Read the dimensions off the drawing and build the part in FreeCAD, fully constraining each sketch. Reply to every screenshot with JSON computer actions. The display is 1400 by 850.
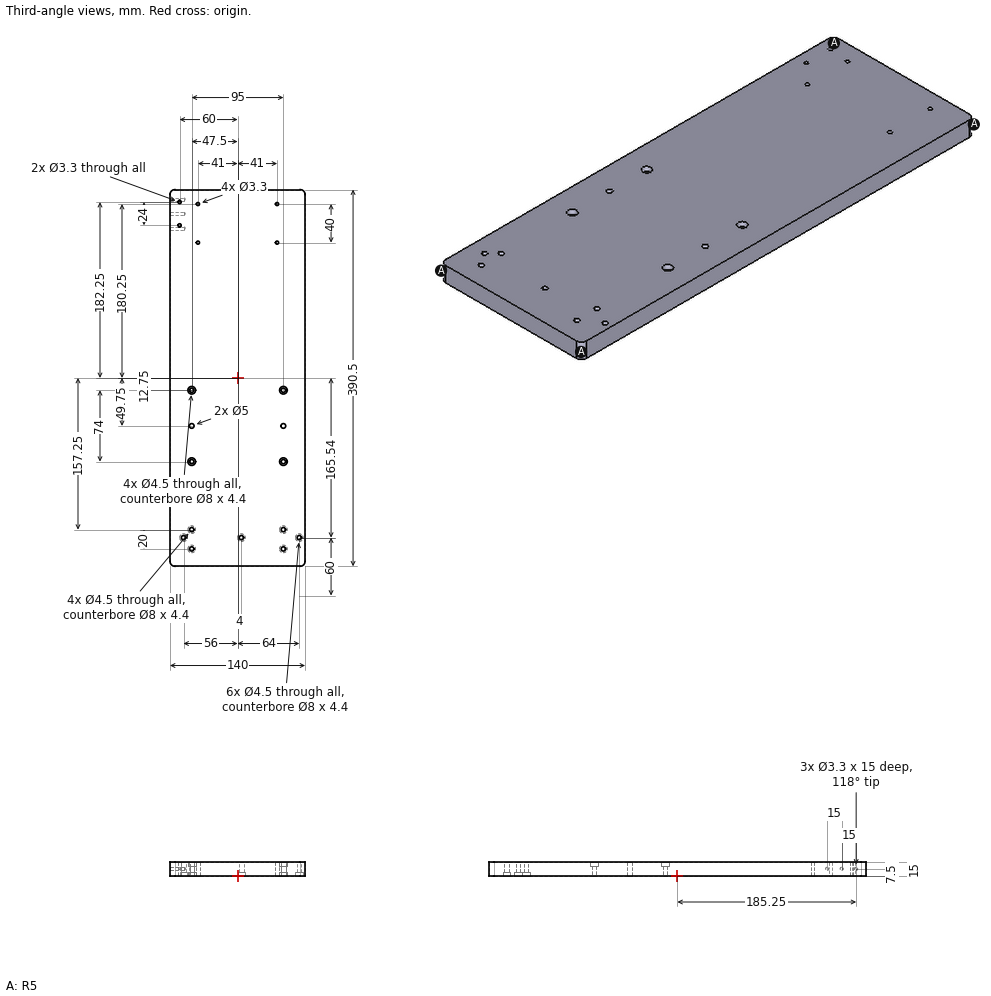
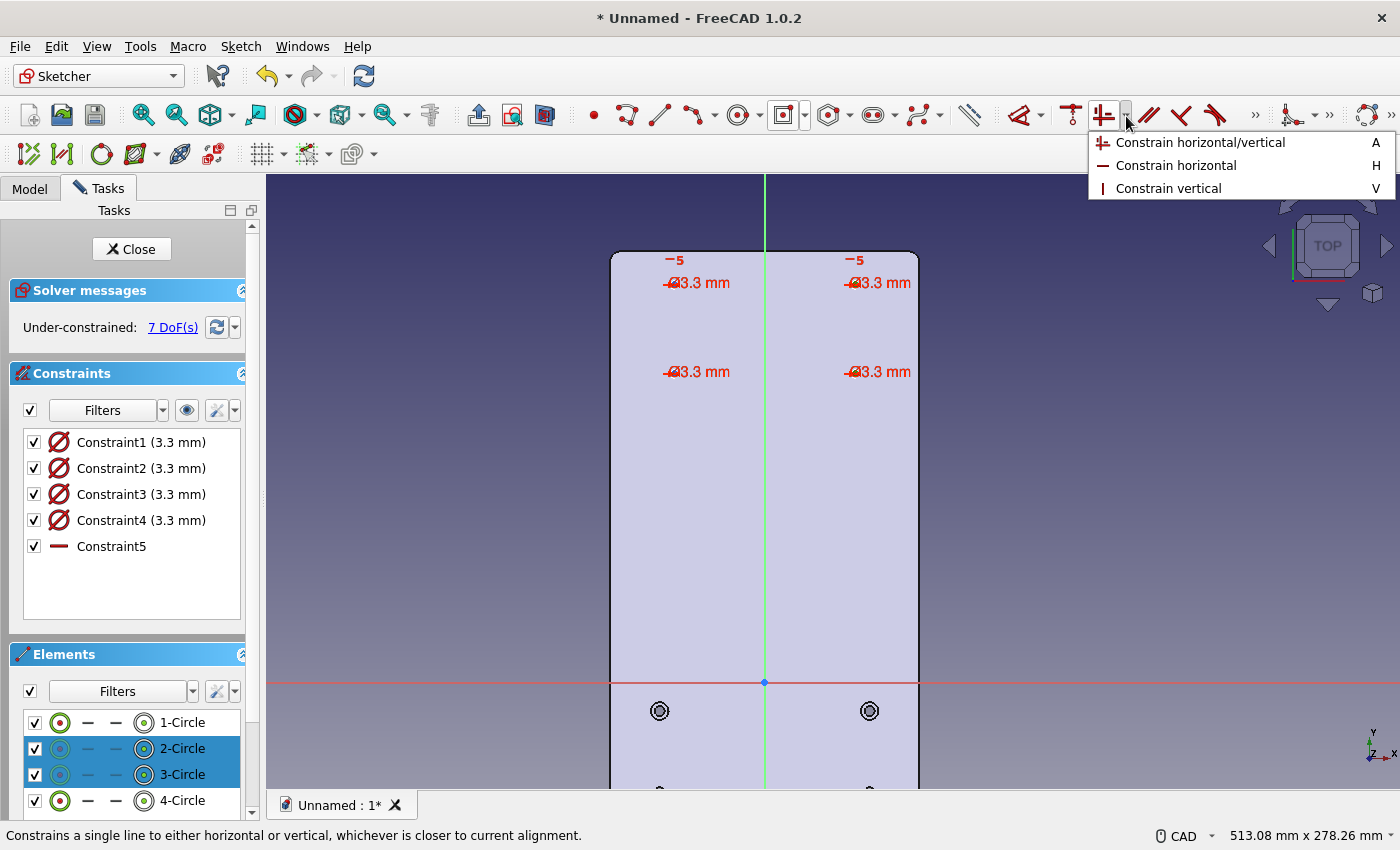
{"action": "left_click", "coordinate": [1242, 188]}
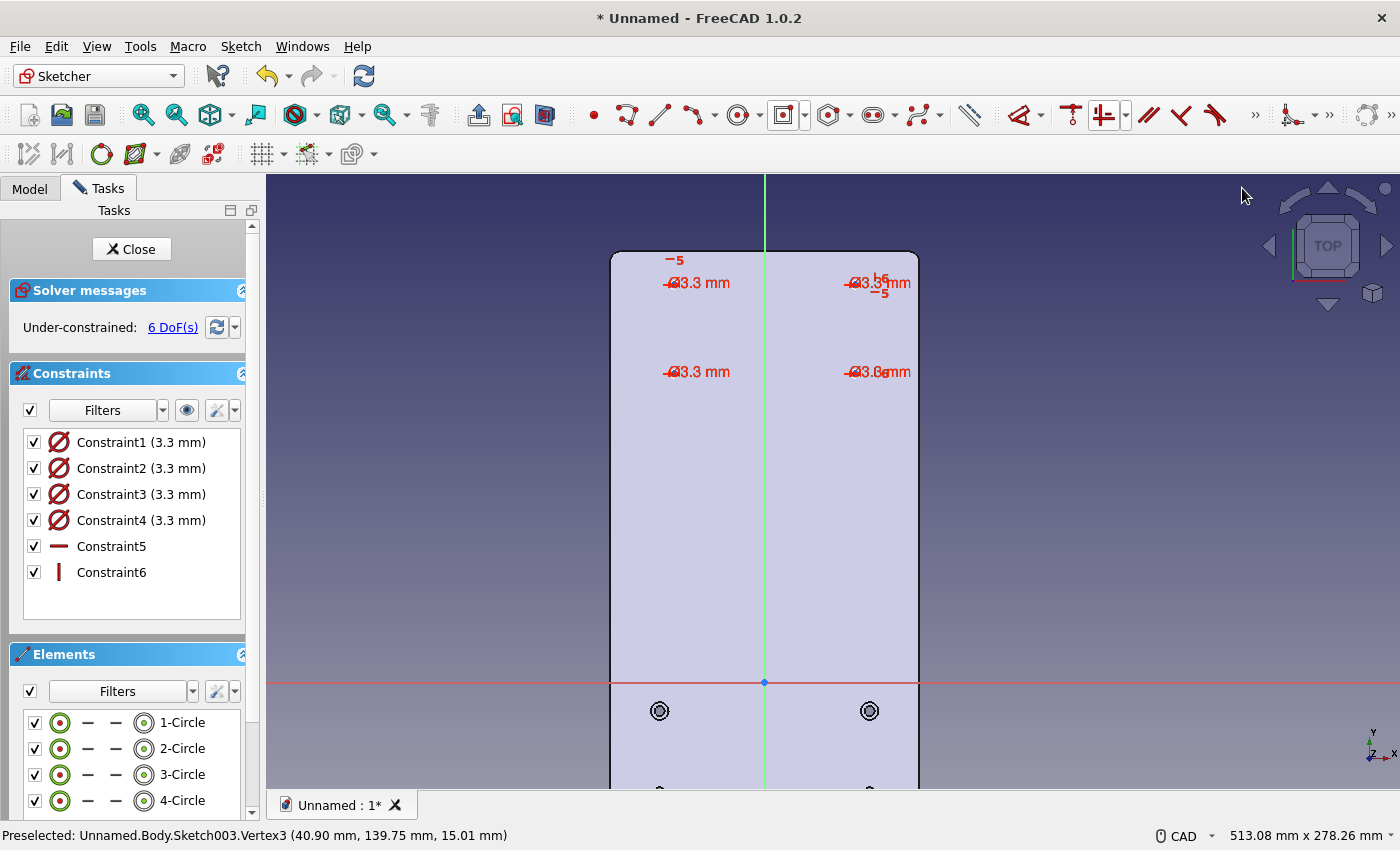
{"action": "left_click", "coordinate": [674, 285]}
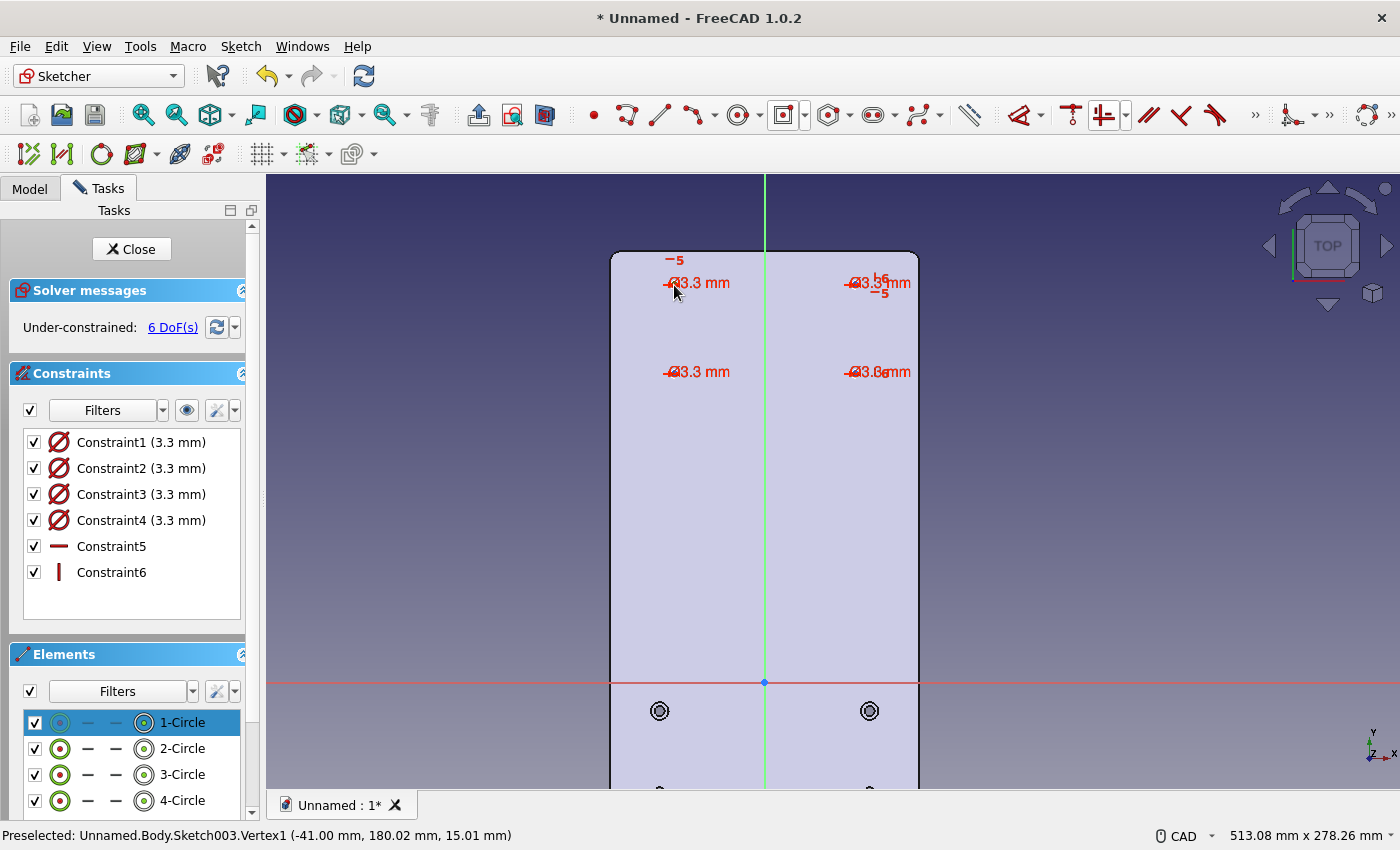
{"action": "left_click", "coordinate": [674, 374]}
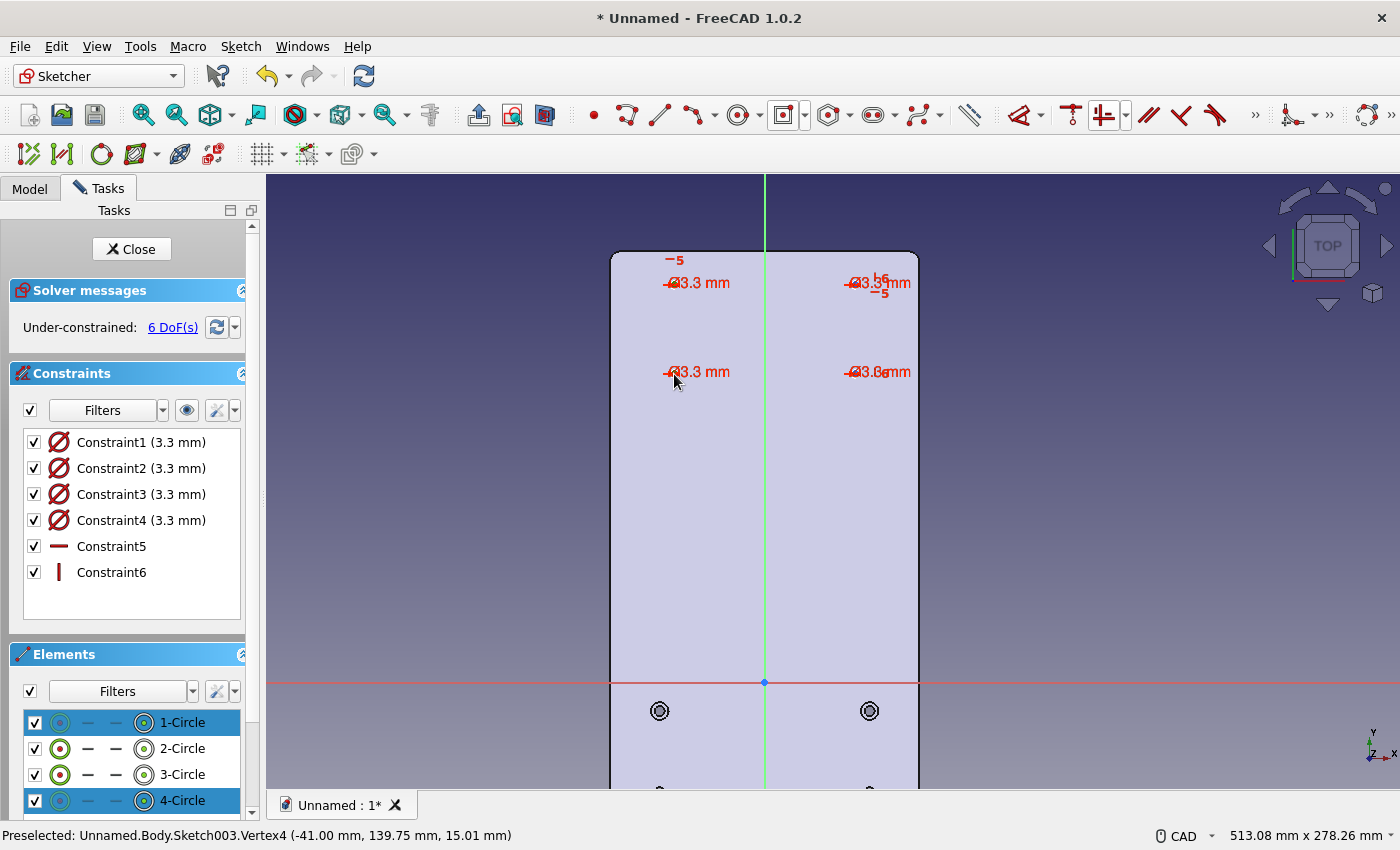
{"action": "left_click", "coordinate": [1126, 116]}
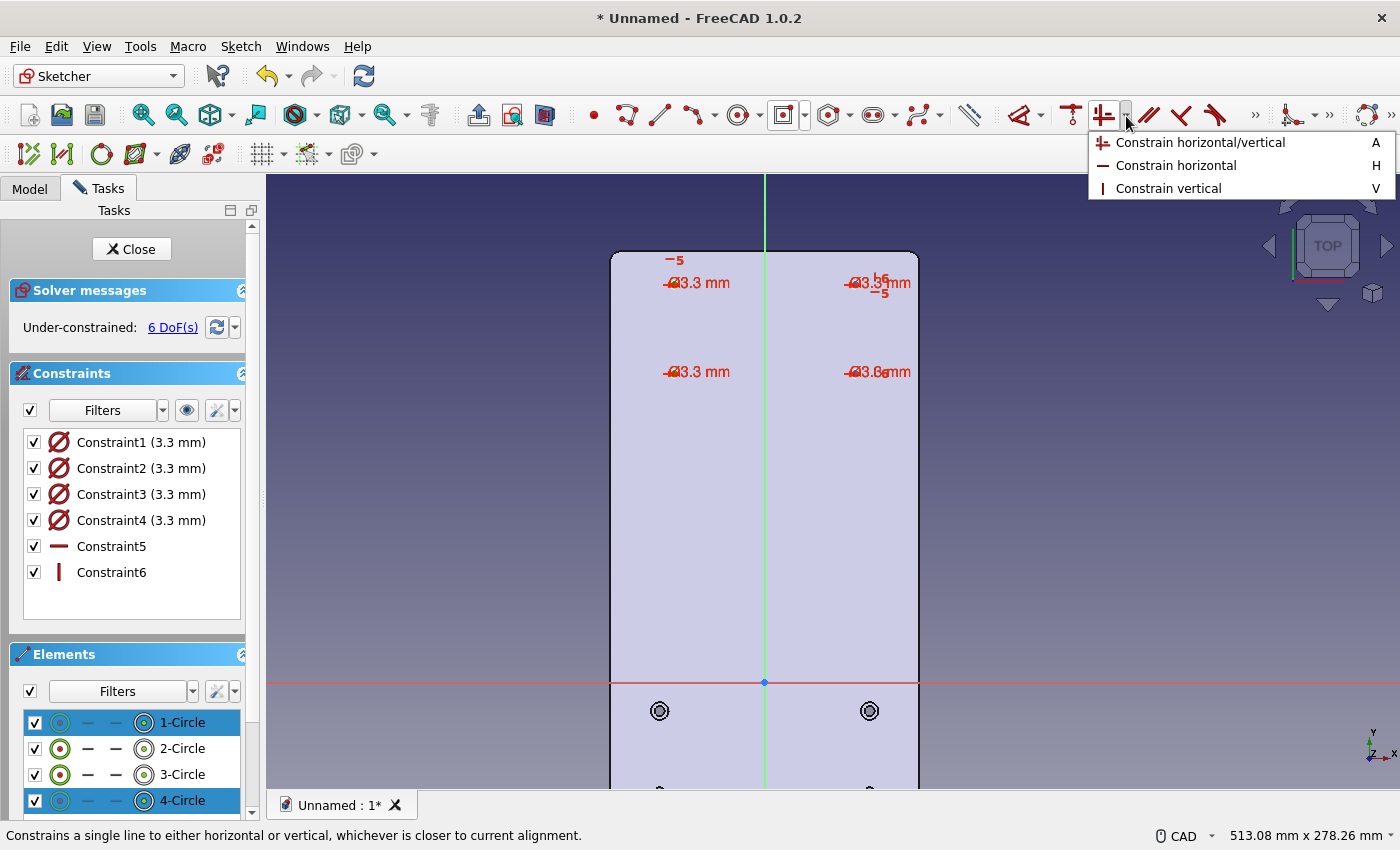
{"action": "left_click", "coordinate": [1242, 188]}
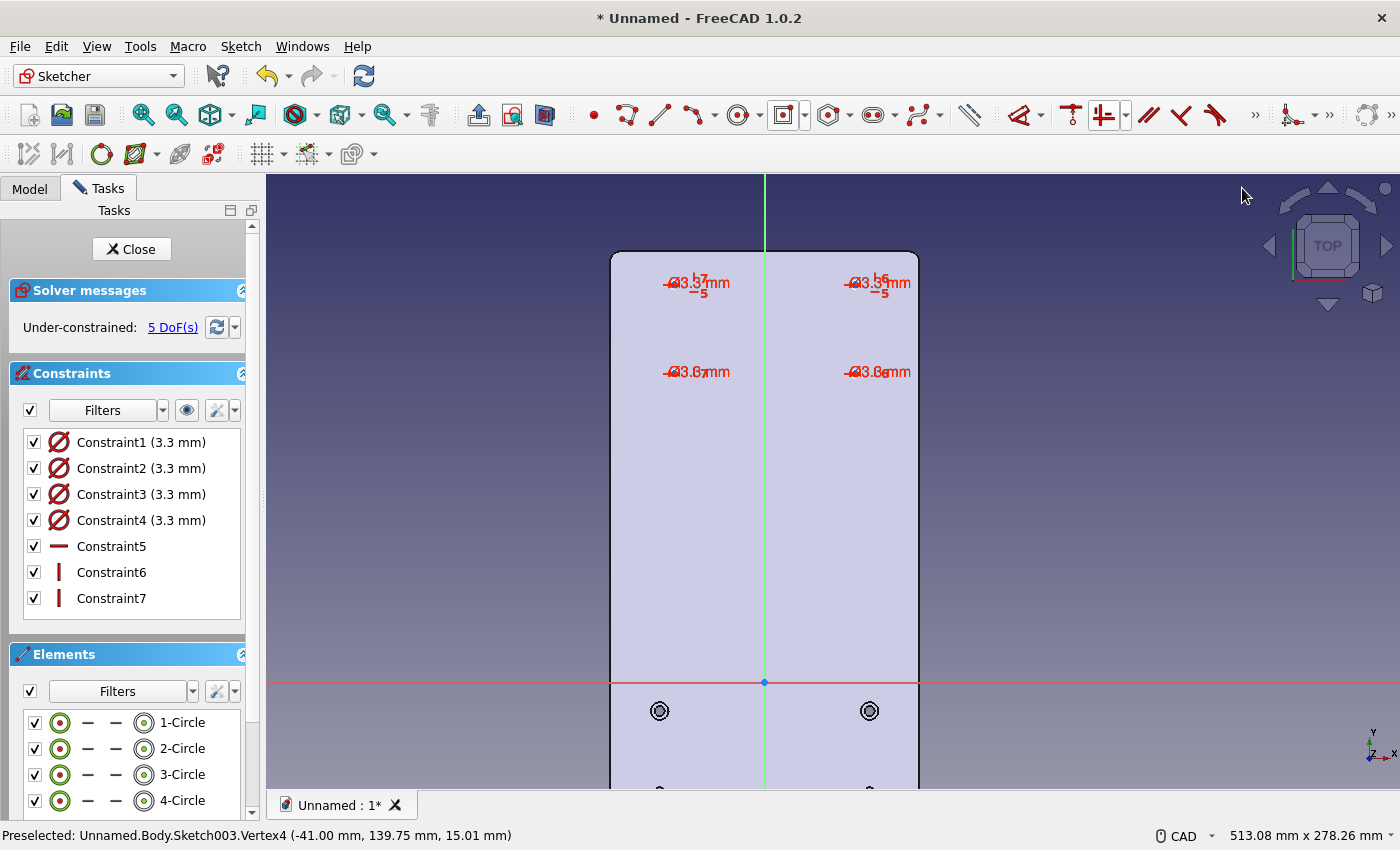
{"action": "left_click", "coordinate": [855, 374]}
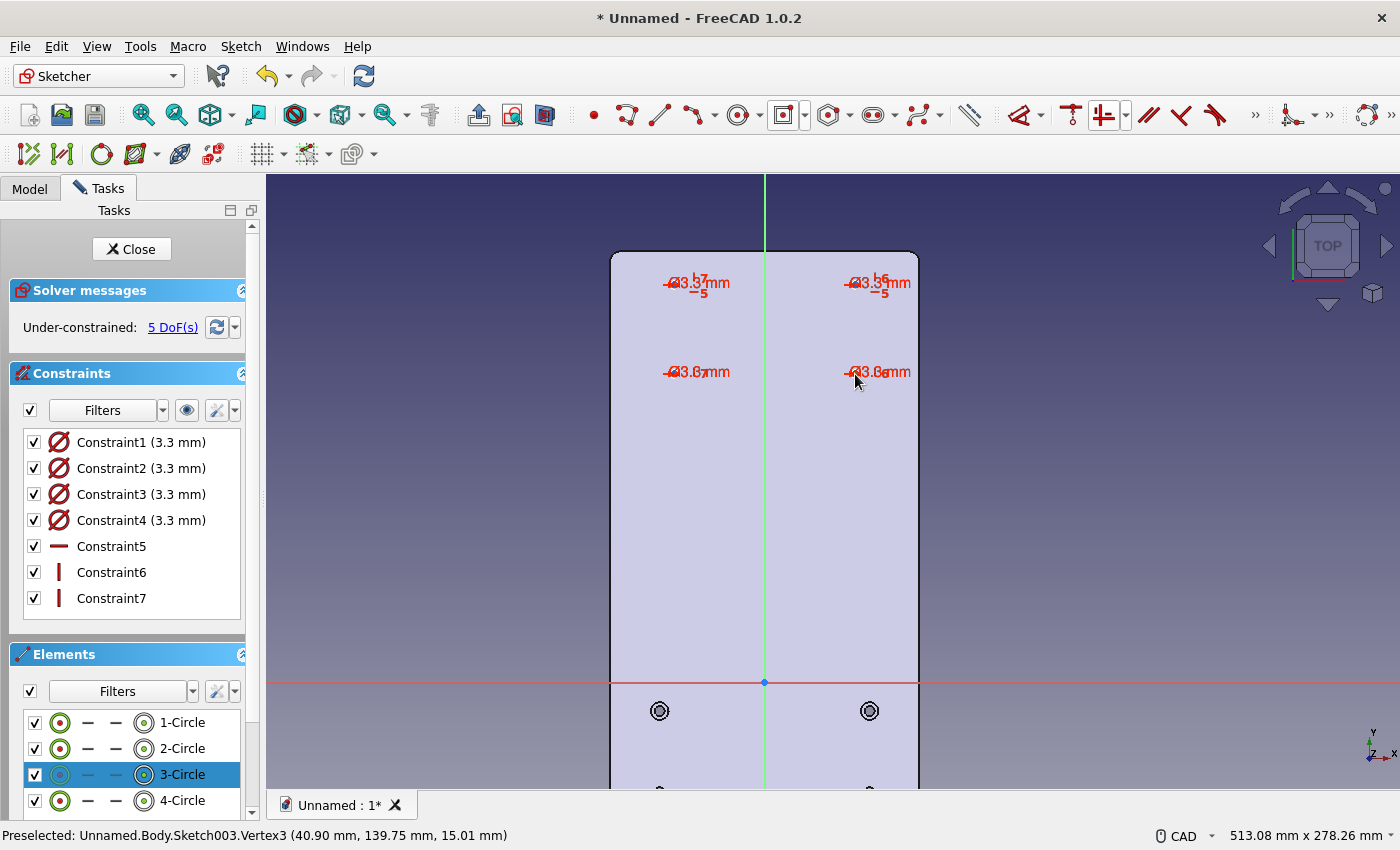
{"action": "left_click", "coordinate": [674, 374]}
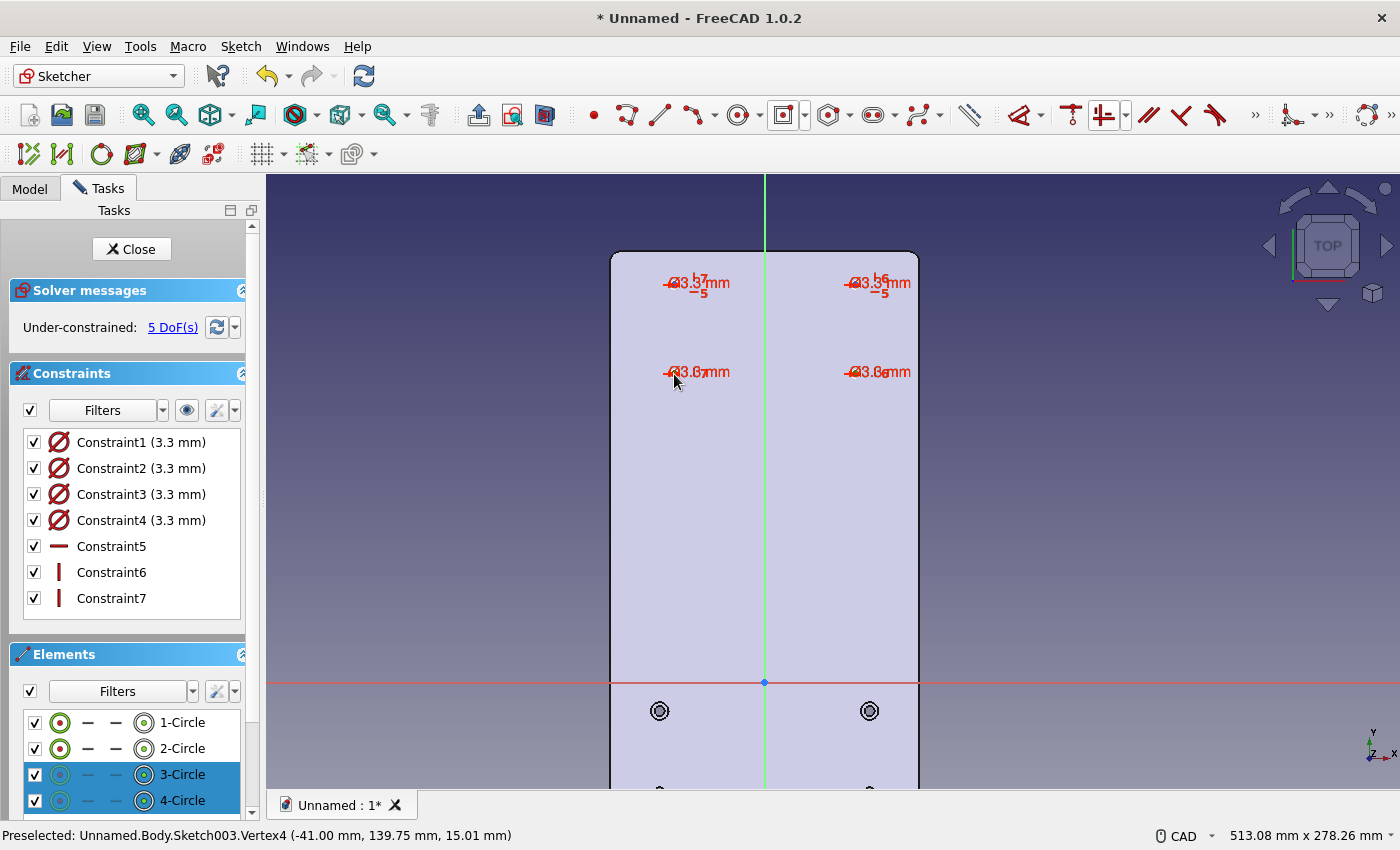
{"action": "key", "text": "h"}